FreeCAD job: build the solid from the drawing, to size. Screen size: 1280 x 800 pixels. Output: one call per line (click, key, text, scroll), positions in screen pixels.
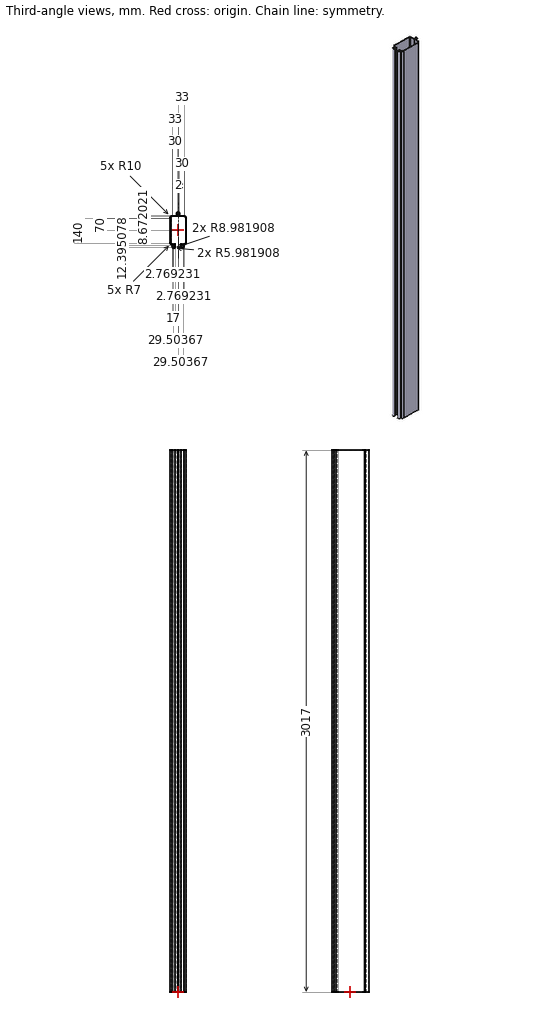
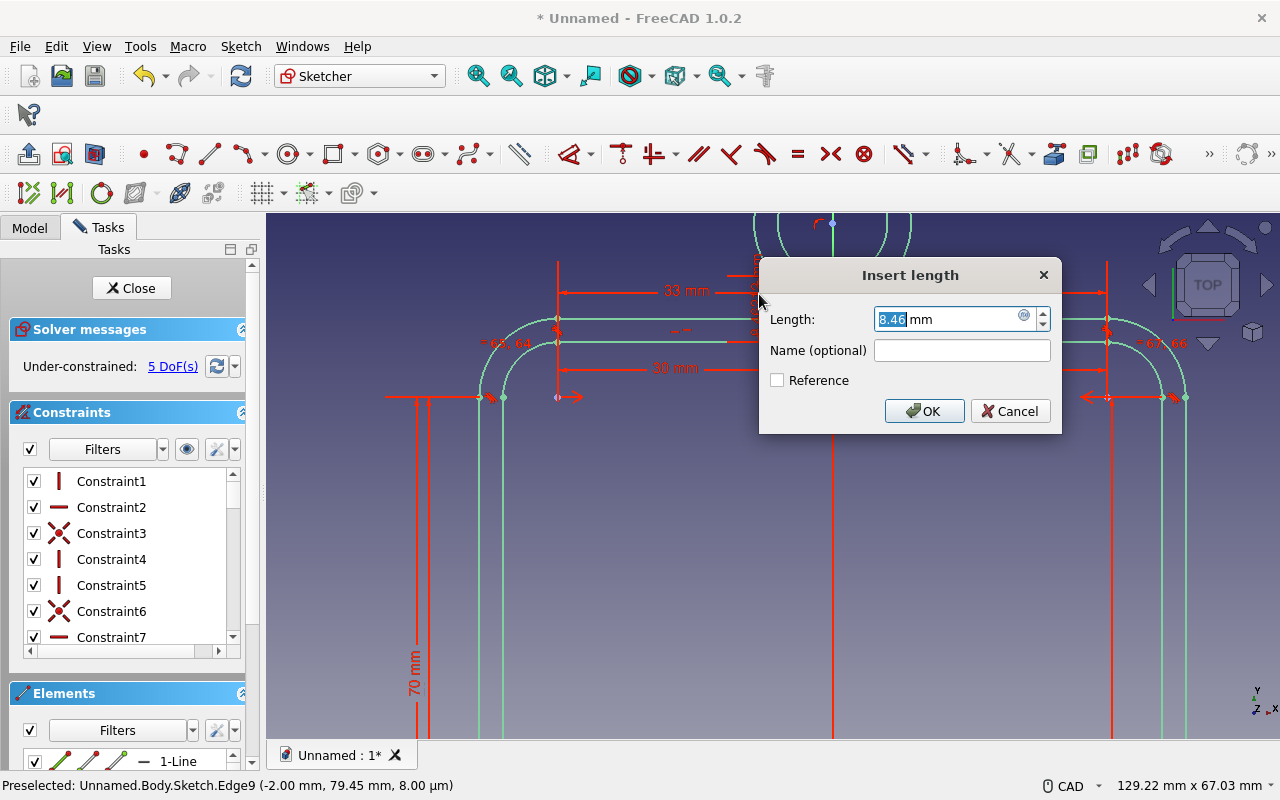
text(8.672021)
key(Return)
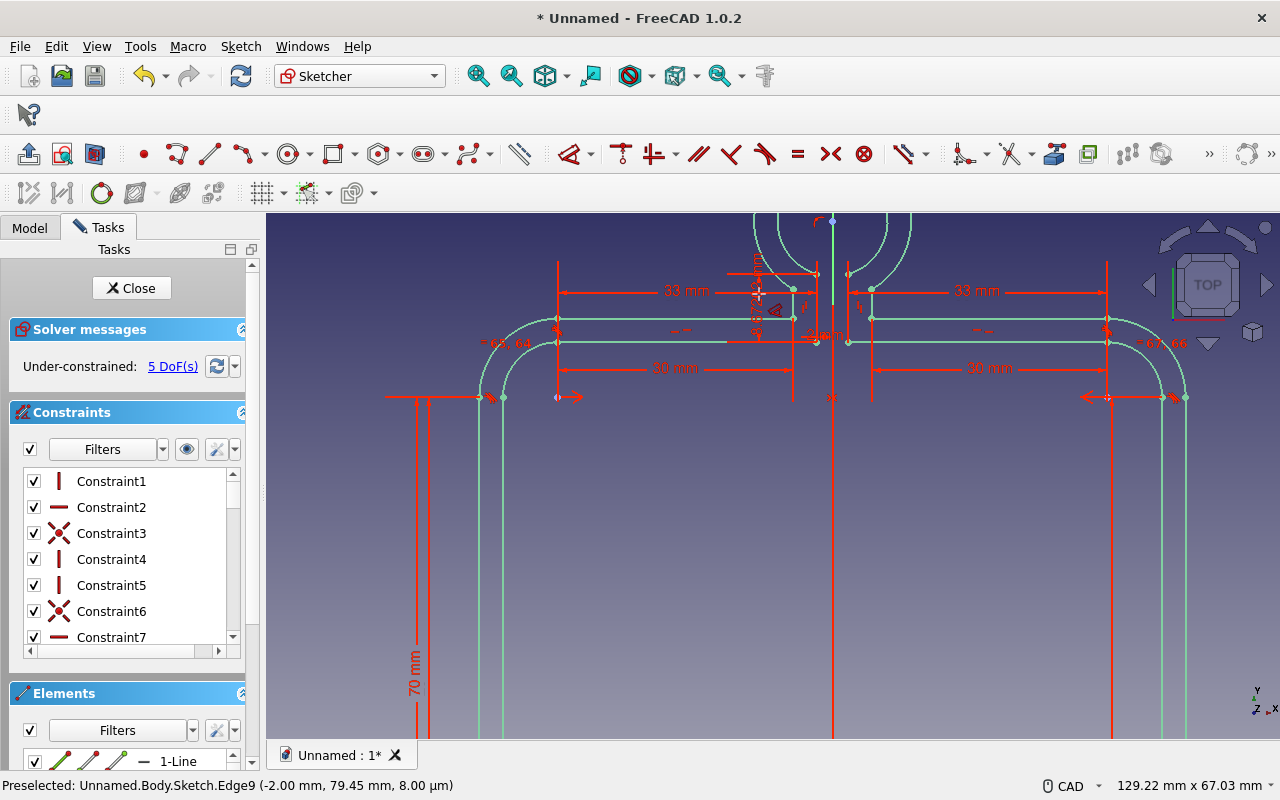
scroll(672, 358, down, 8)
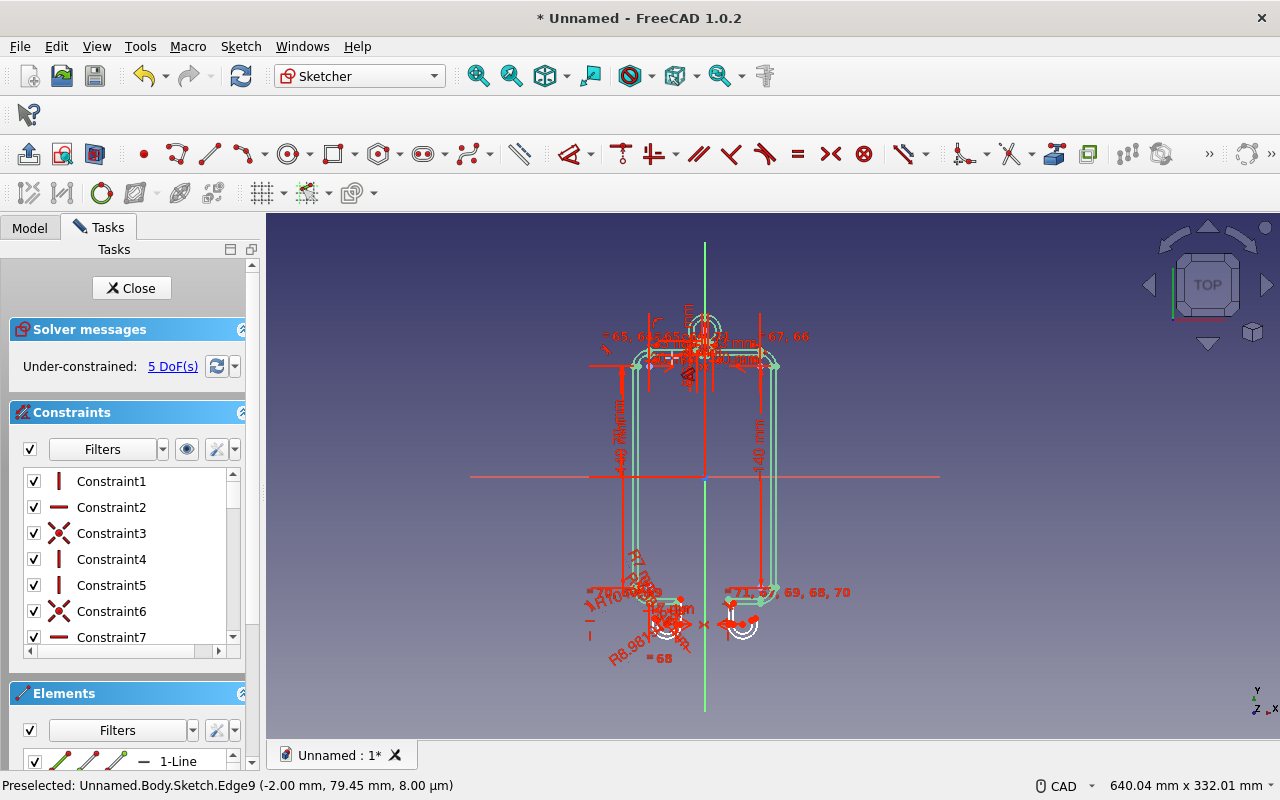
scroll(676, 610, up, 6)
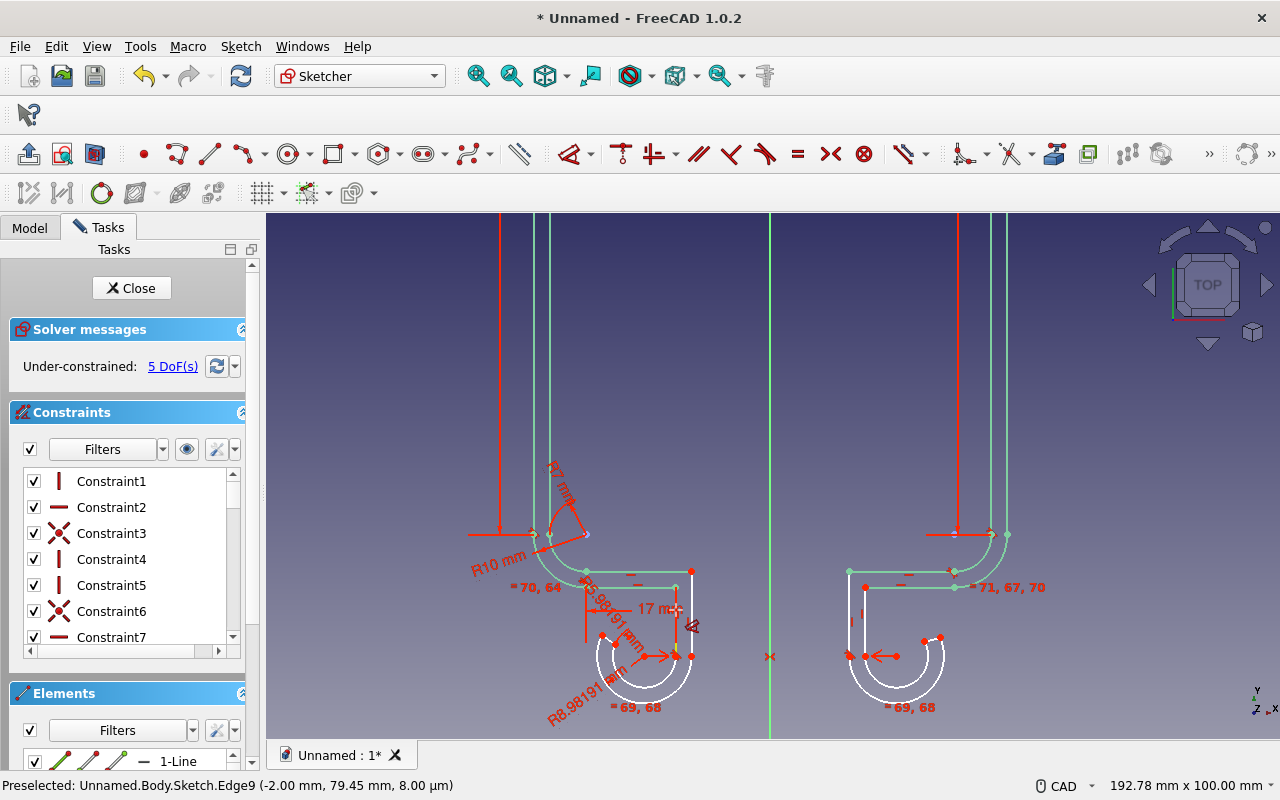
click(676, 608)
click(642, 638)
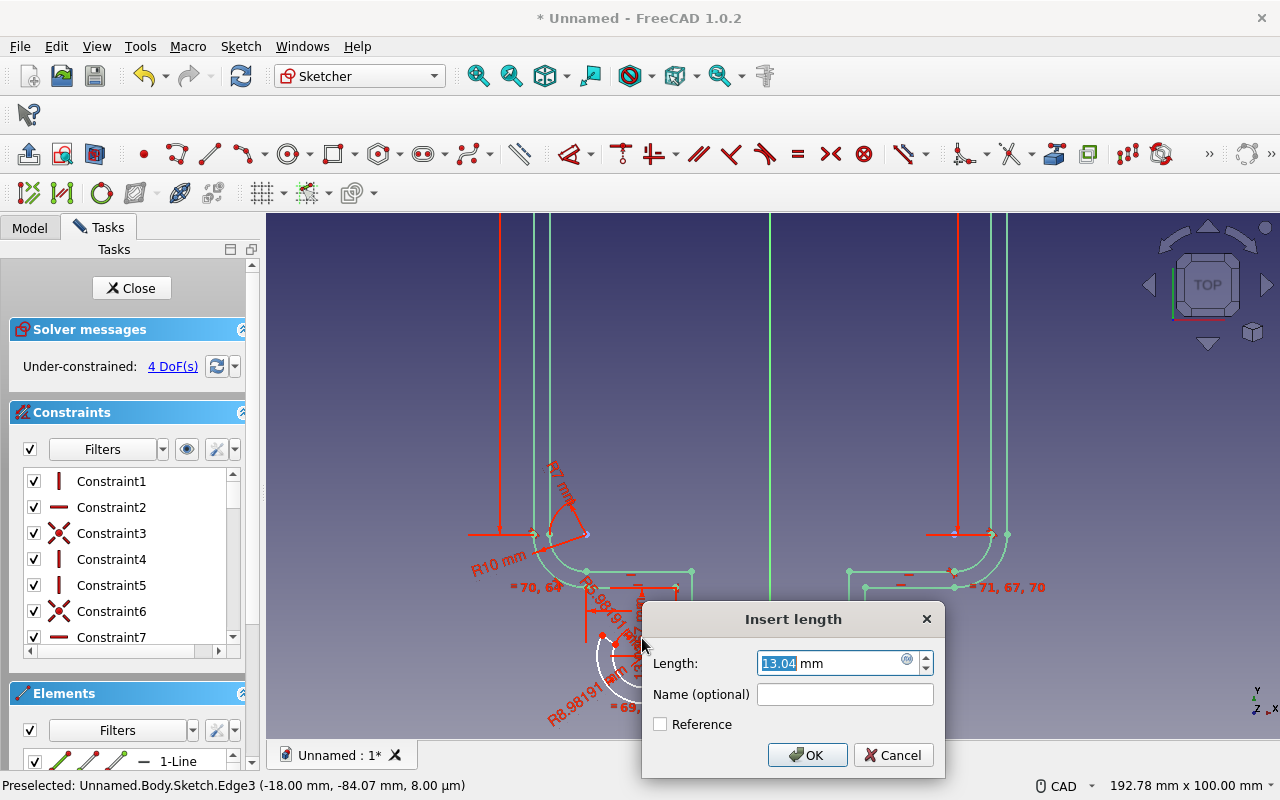
text(12.395078)
key(Return)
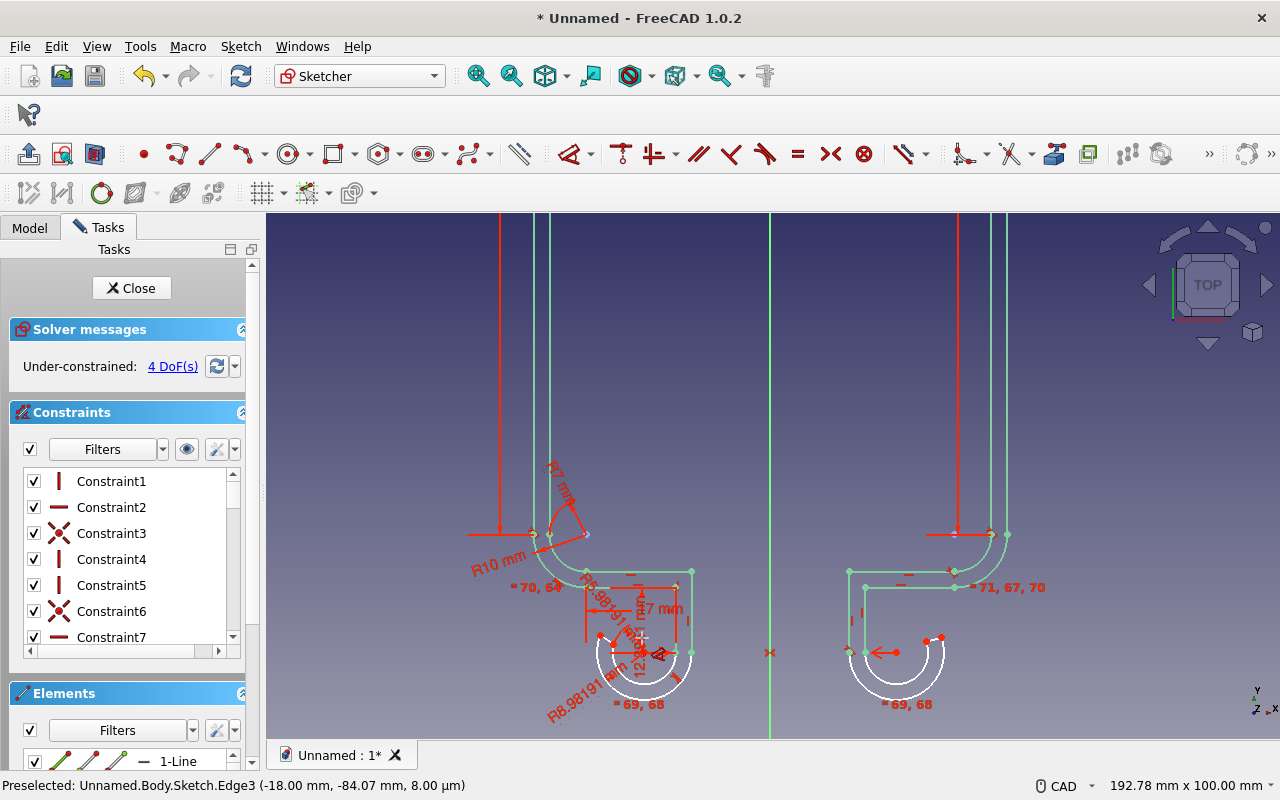
click(614, 645)
click(728, 679)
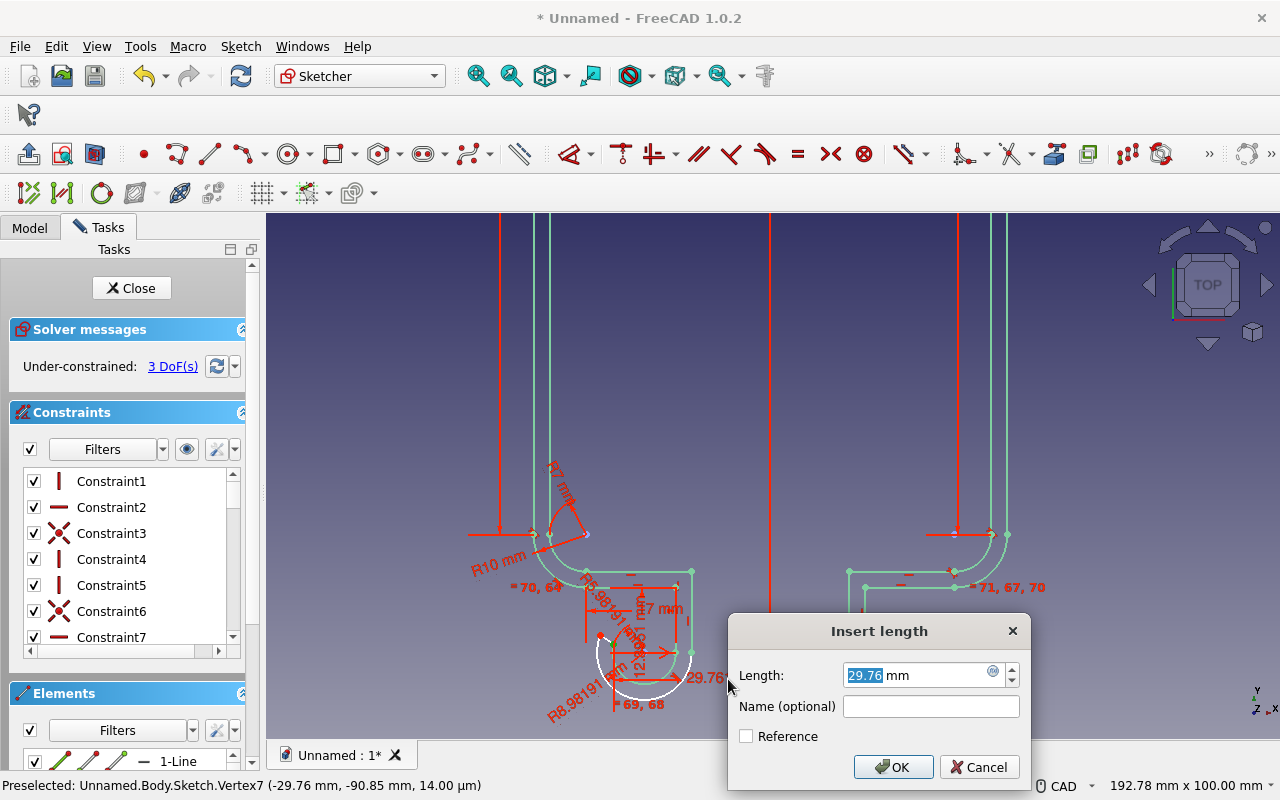
text(29.50367)
key(Return)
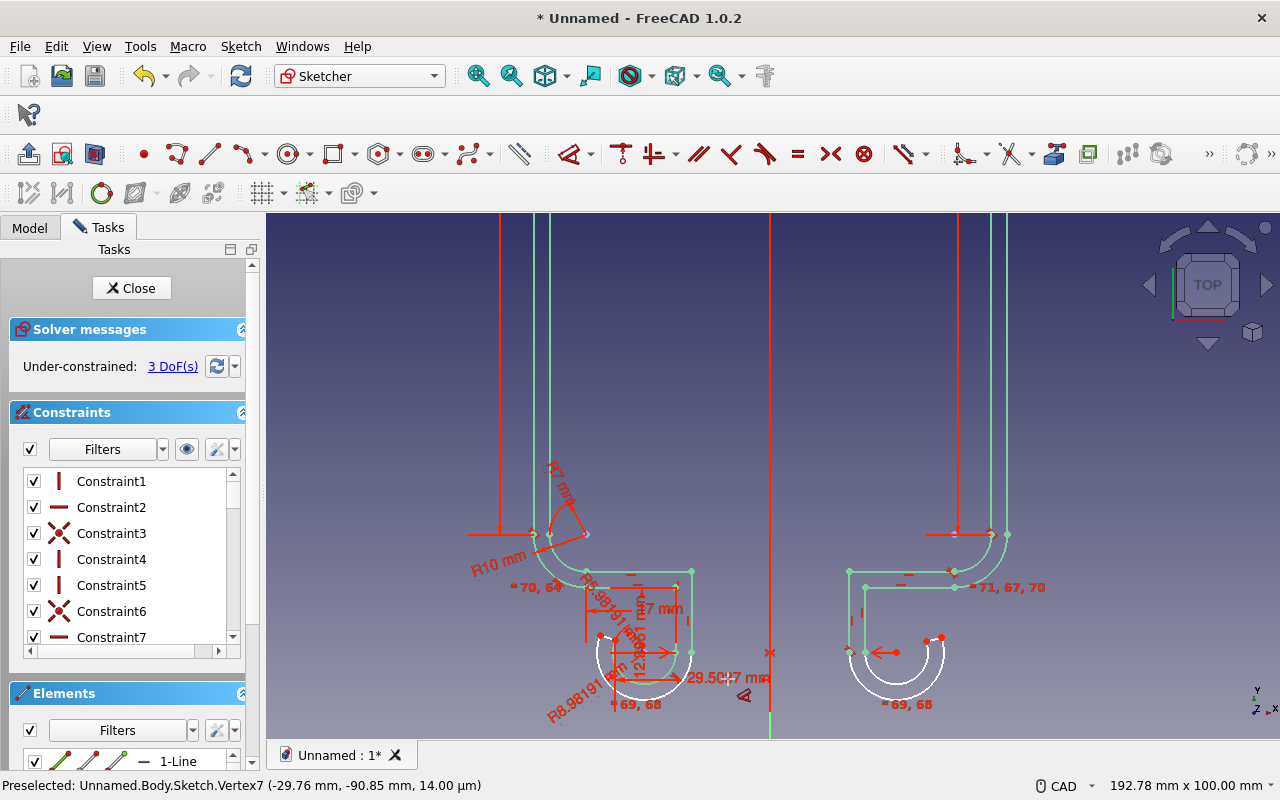
click(926, 642)
click(813, 676)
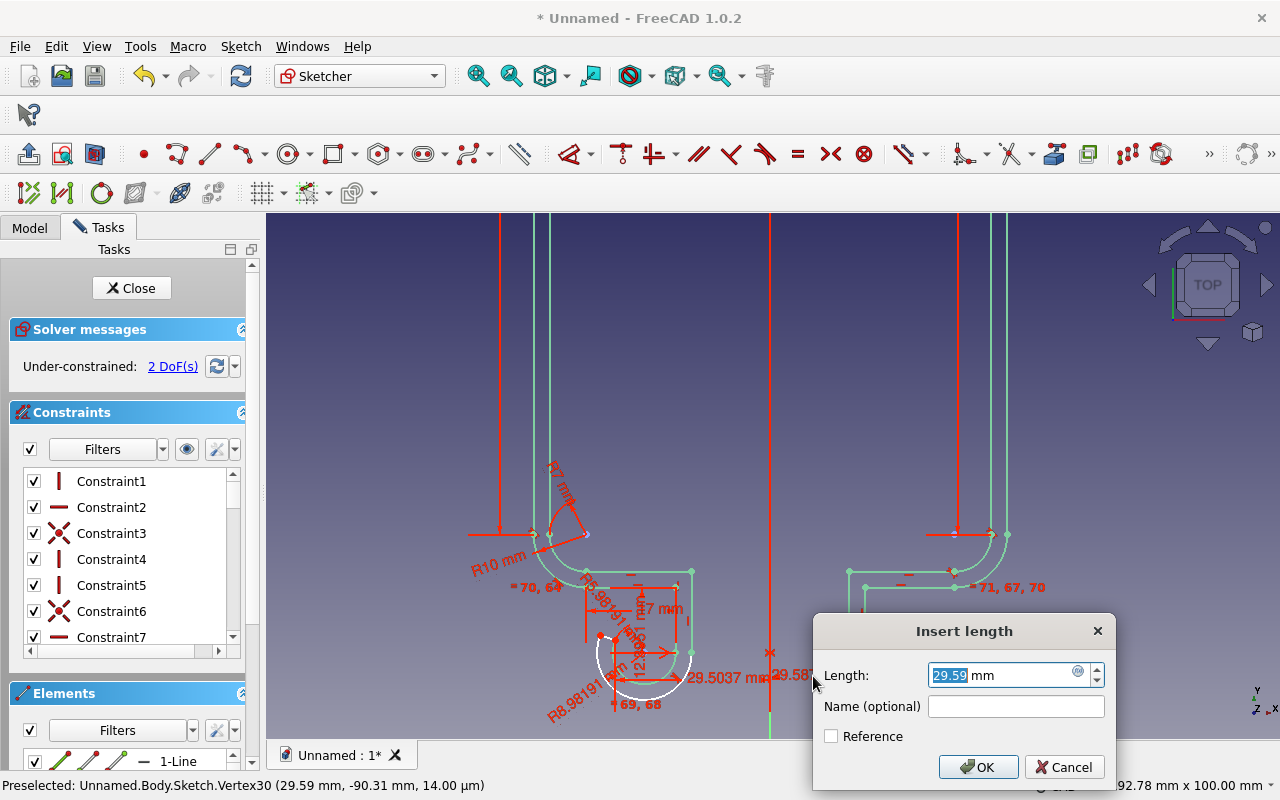
text(29.50367)
key(Return)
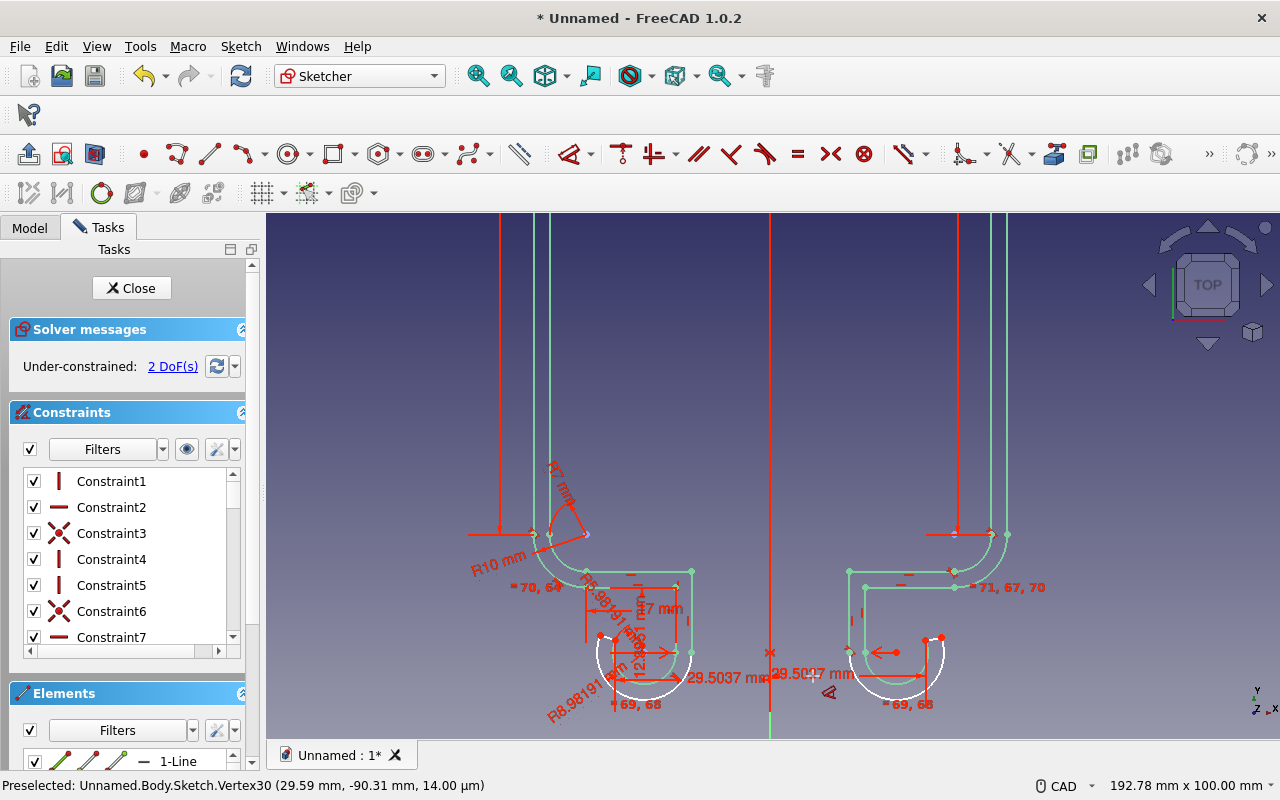
scroll(608, 638, up, 6)